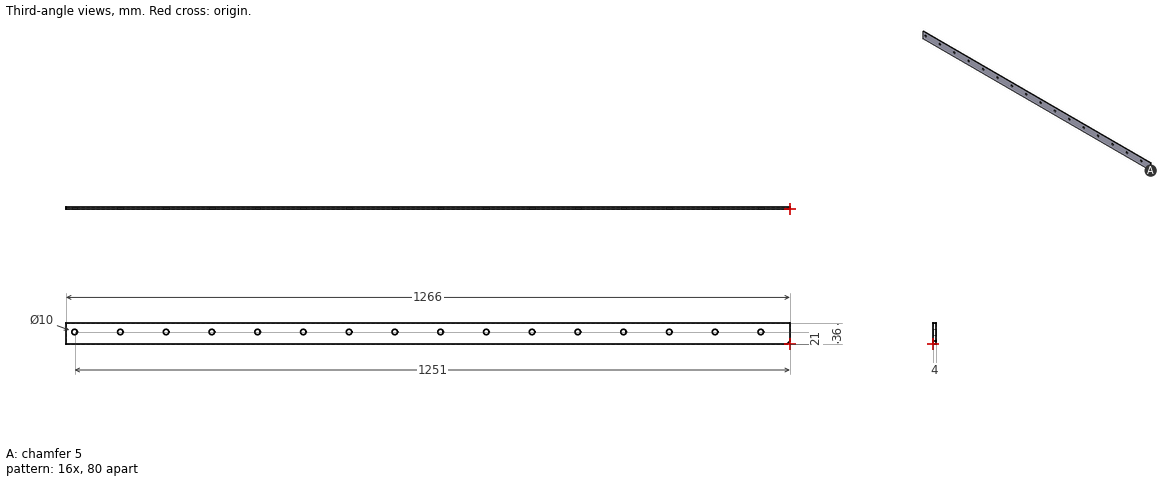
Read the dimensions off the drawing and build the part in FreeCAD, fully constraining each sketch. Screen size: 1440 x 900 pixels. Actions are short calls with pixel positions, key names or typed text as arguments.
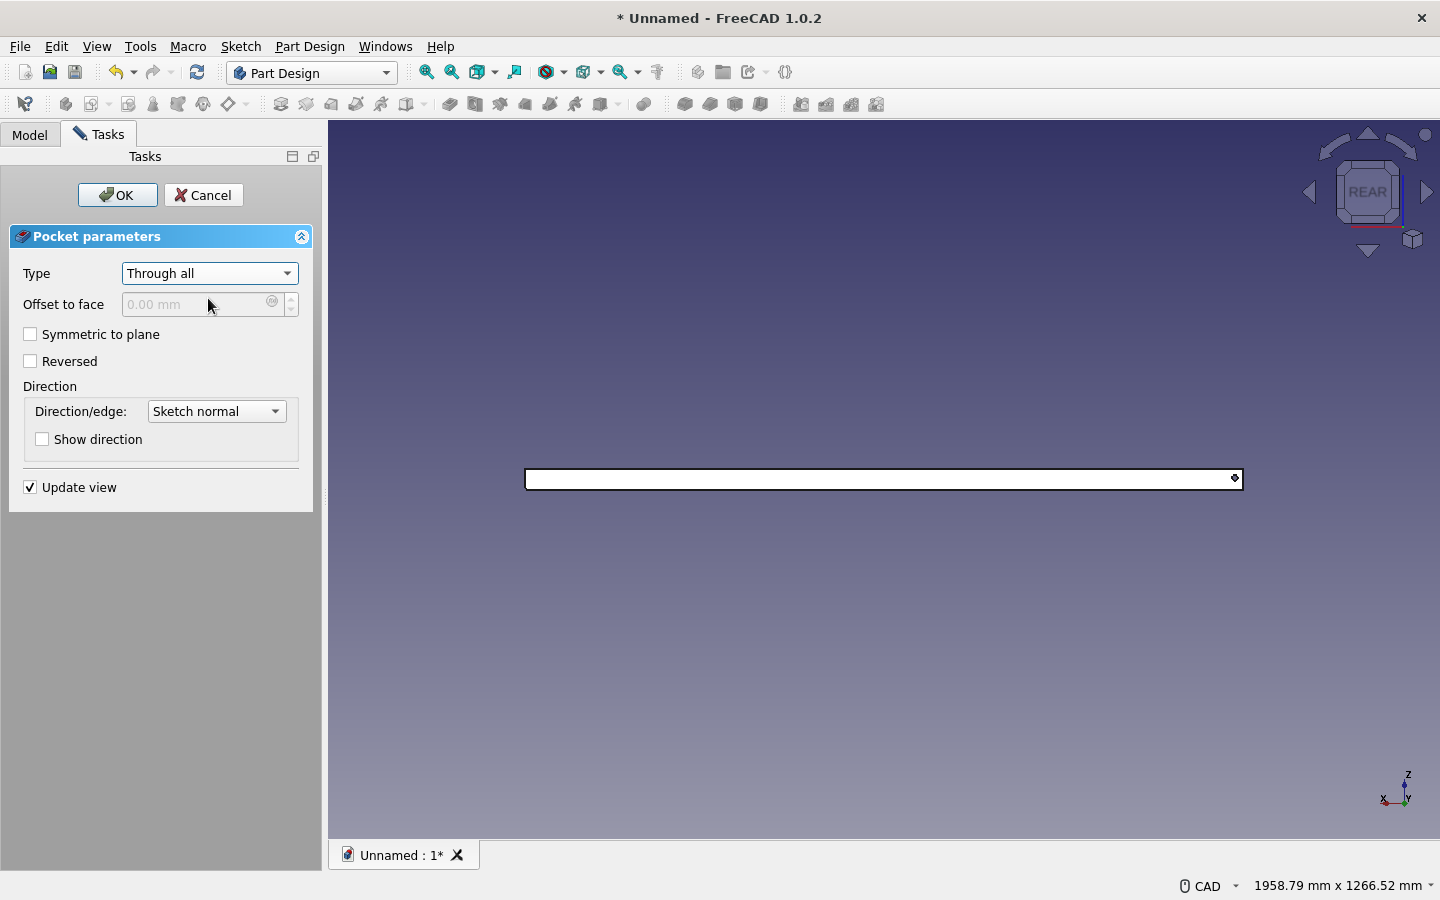
click(118, 195)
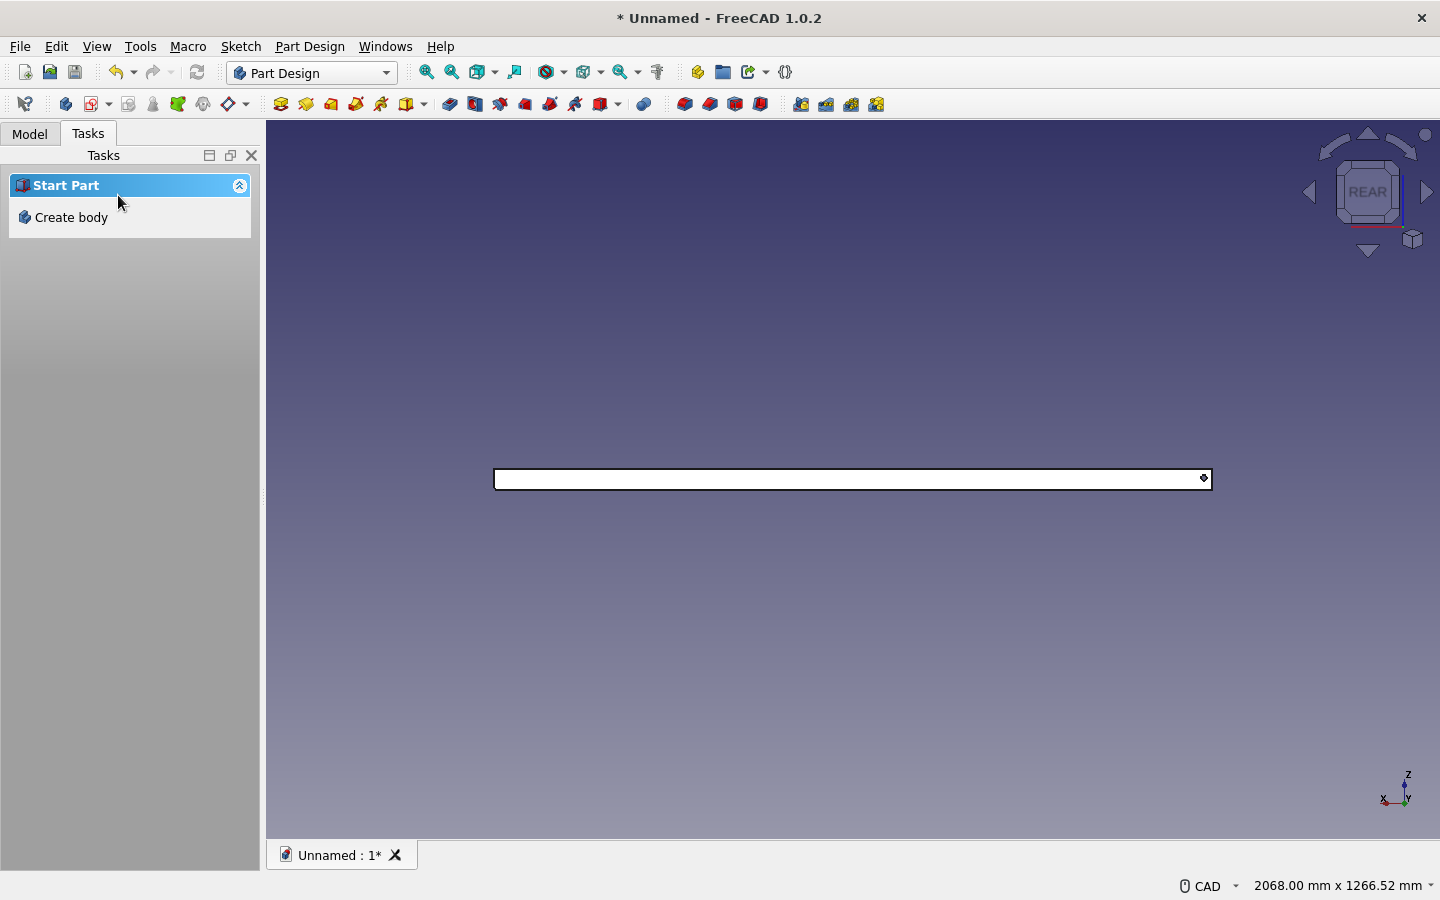
click(30, 134)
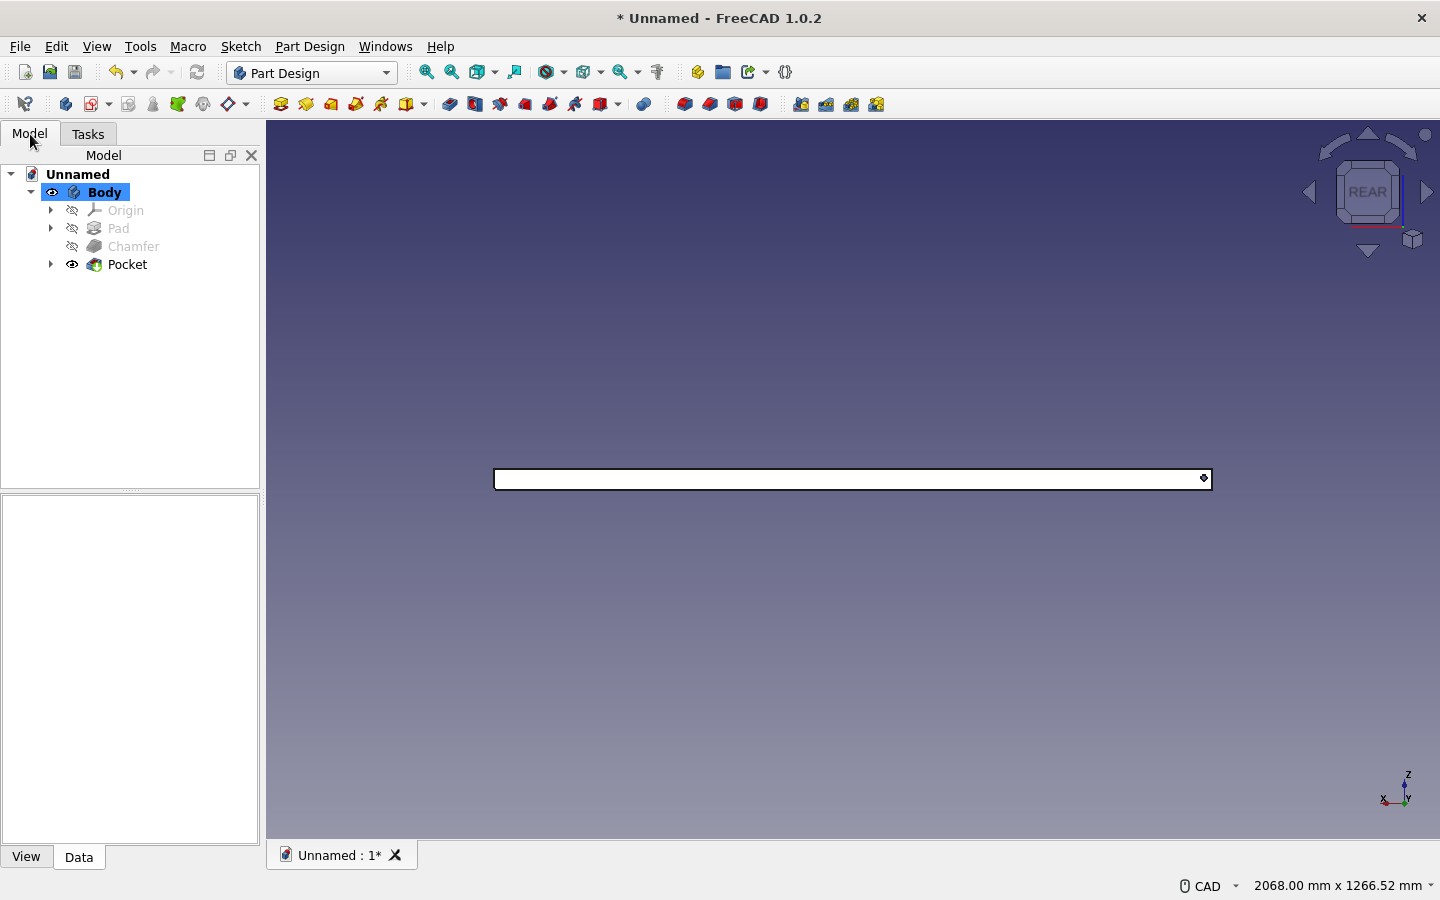
click(117, 264)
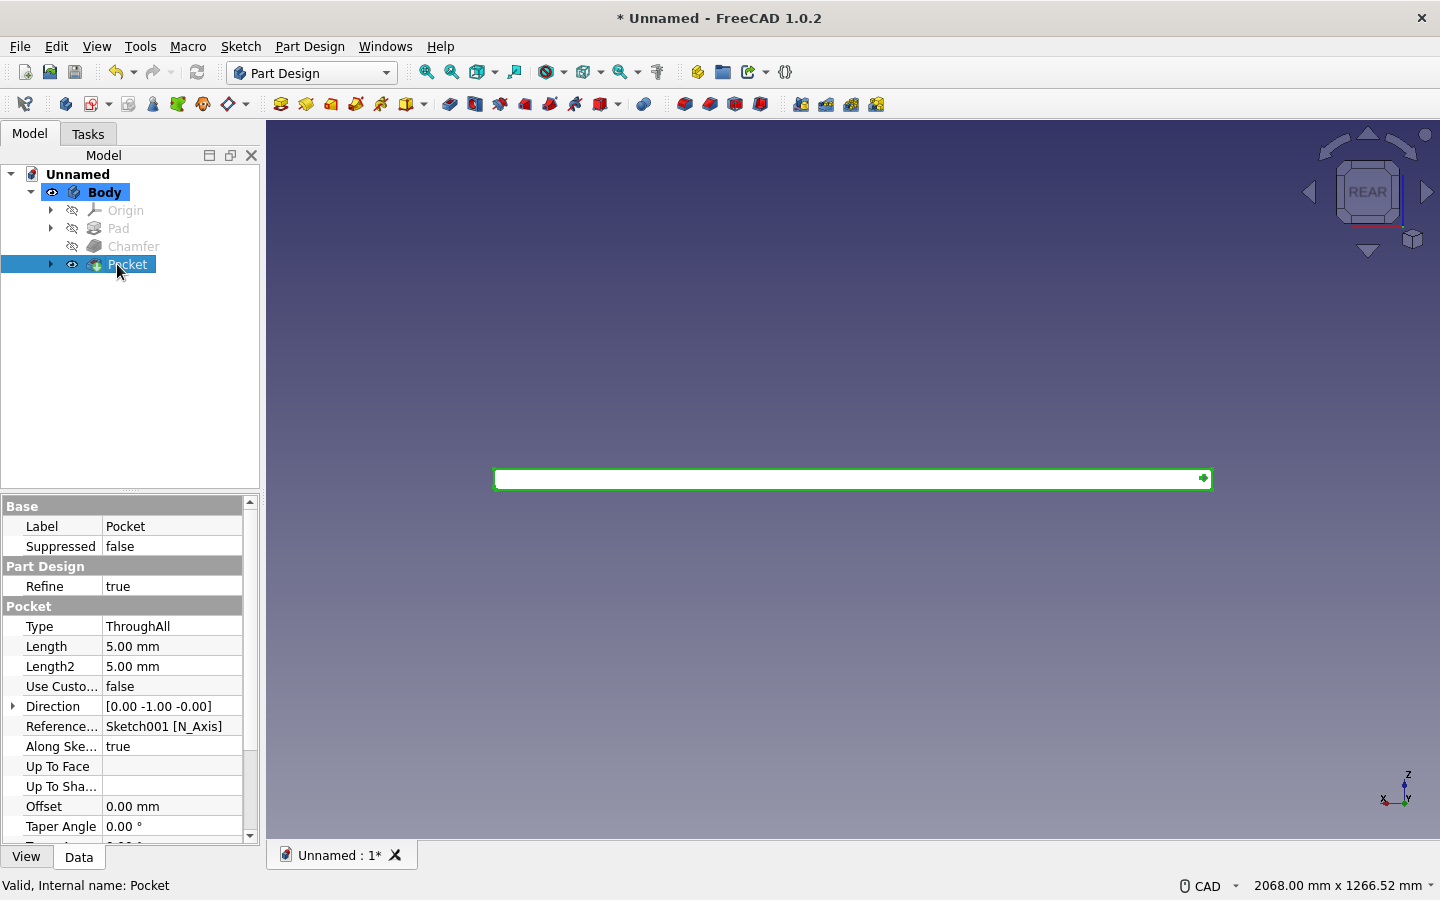
click(826, 104)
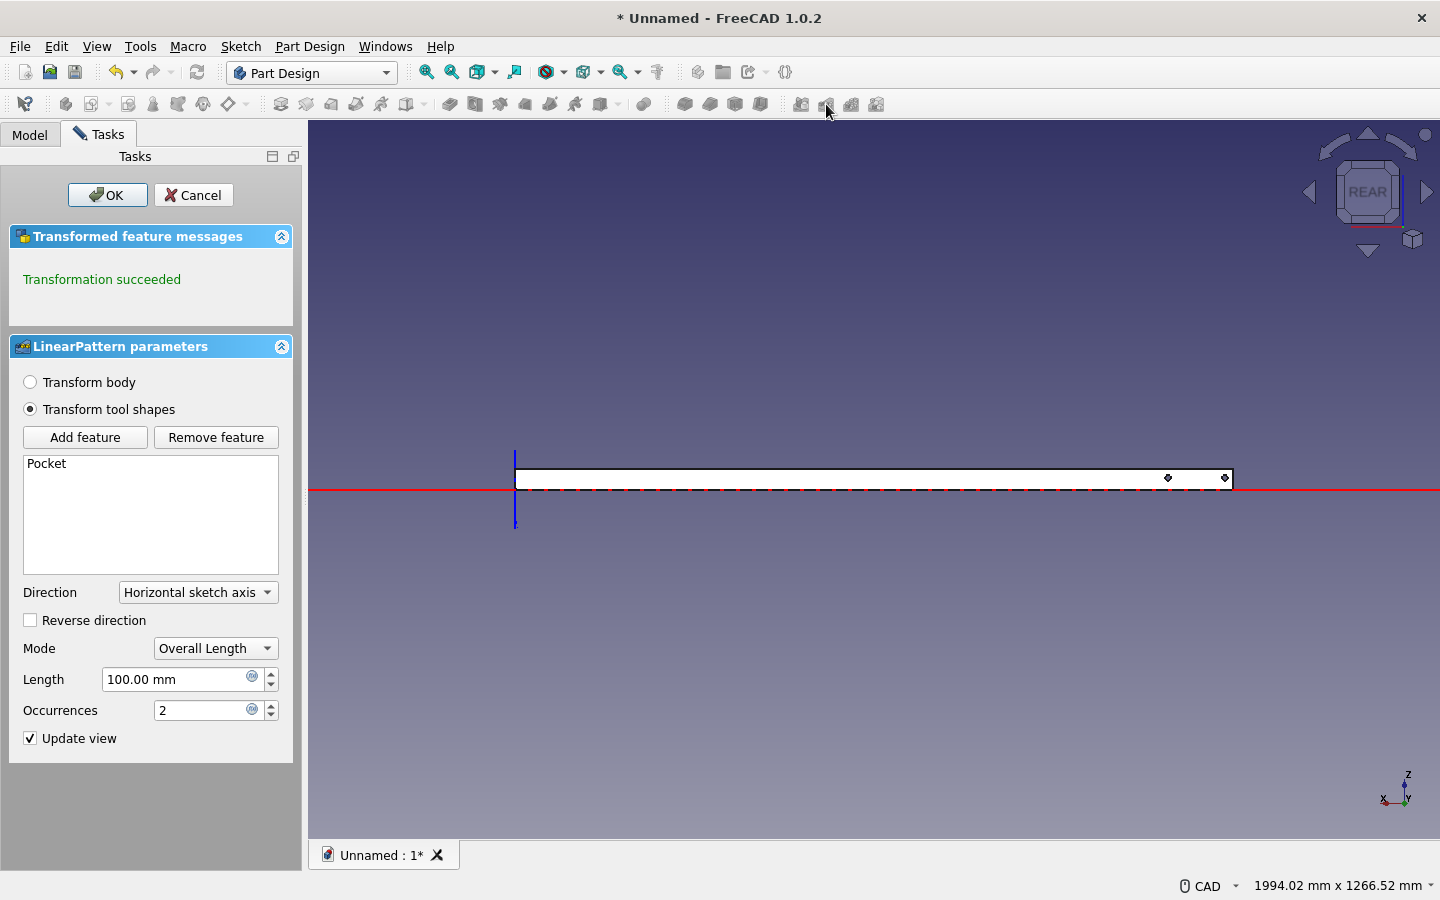
click(199, 592)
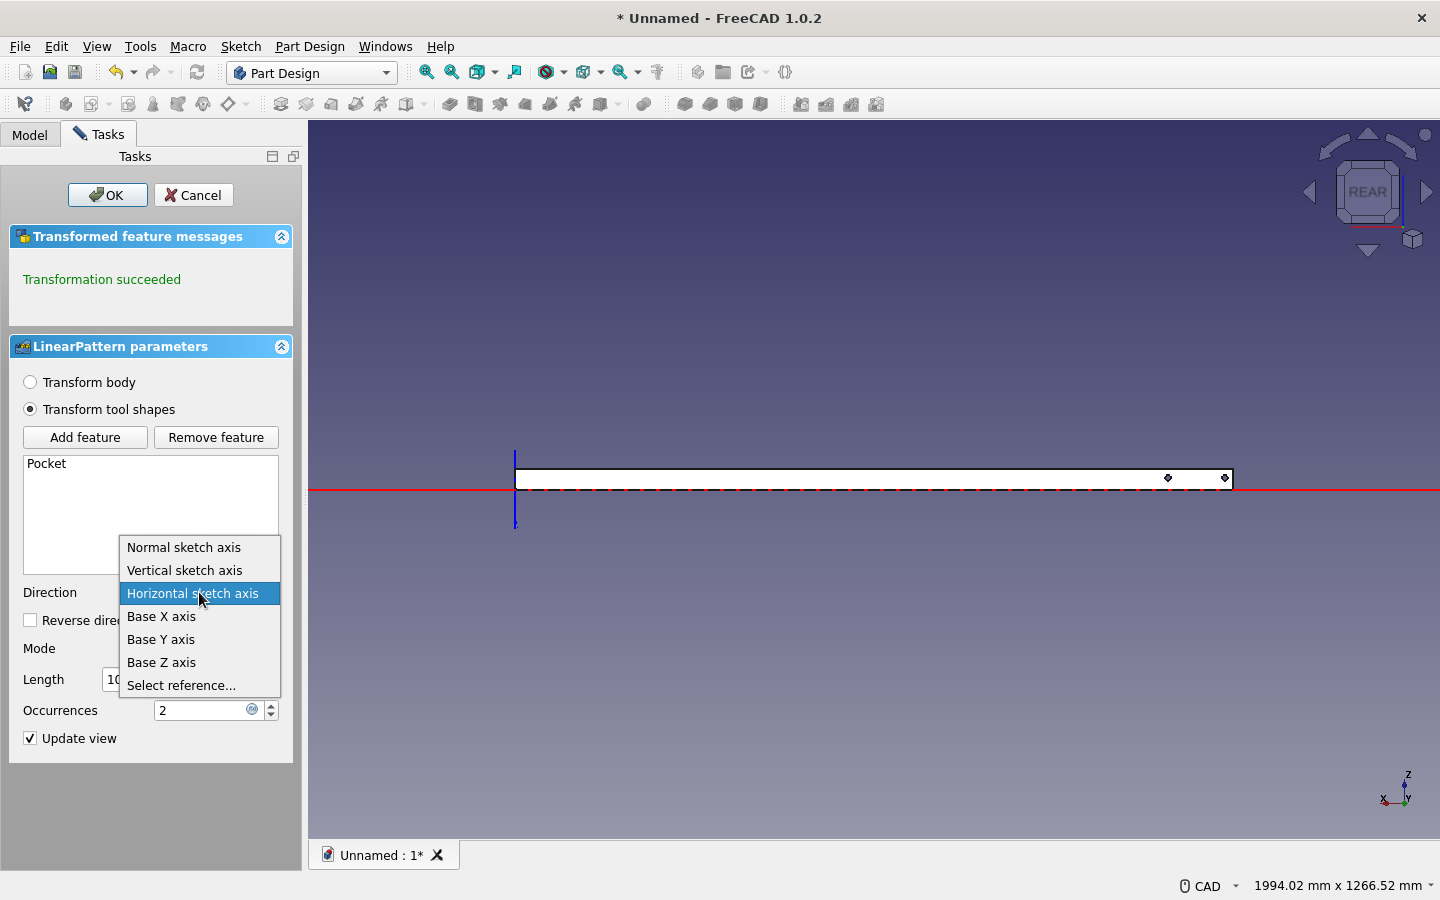
click(198, 616)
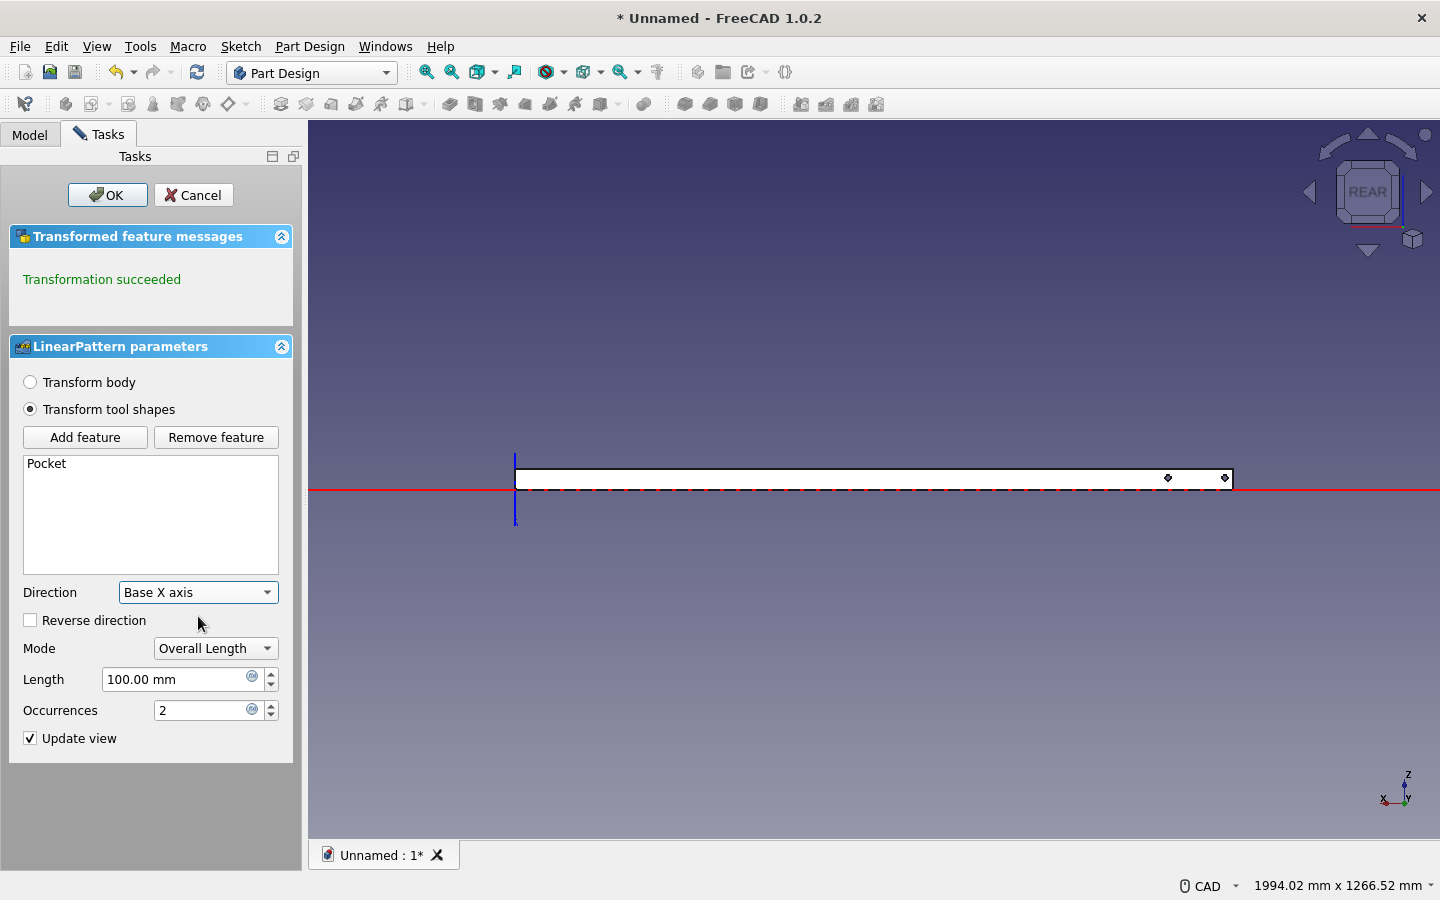
click(216, 648)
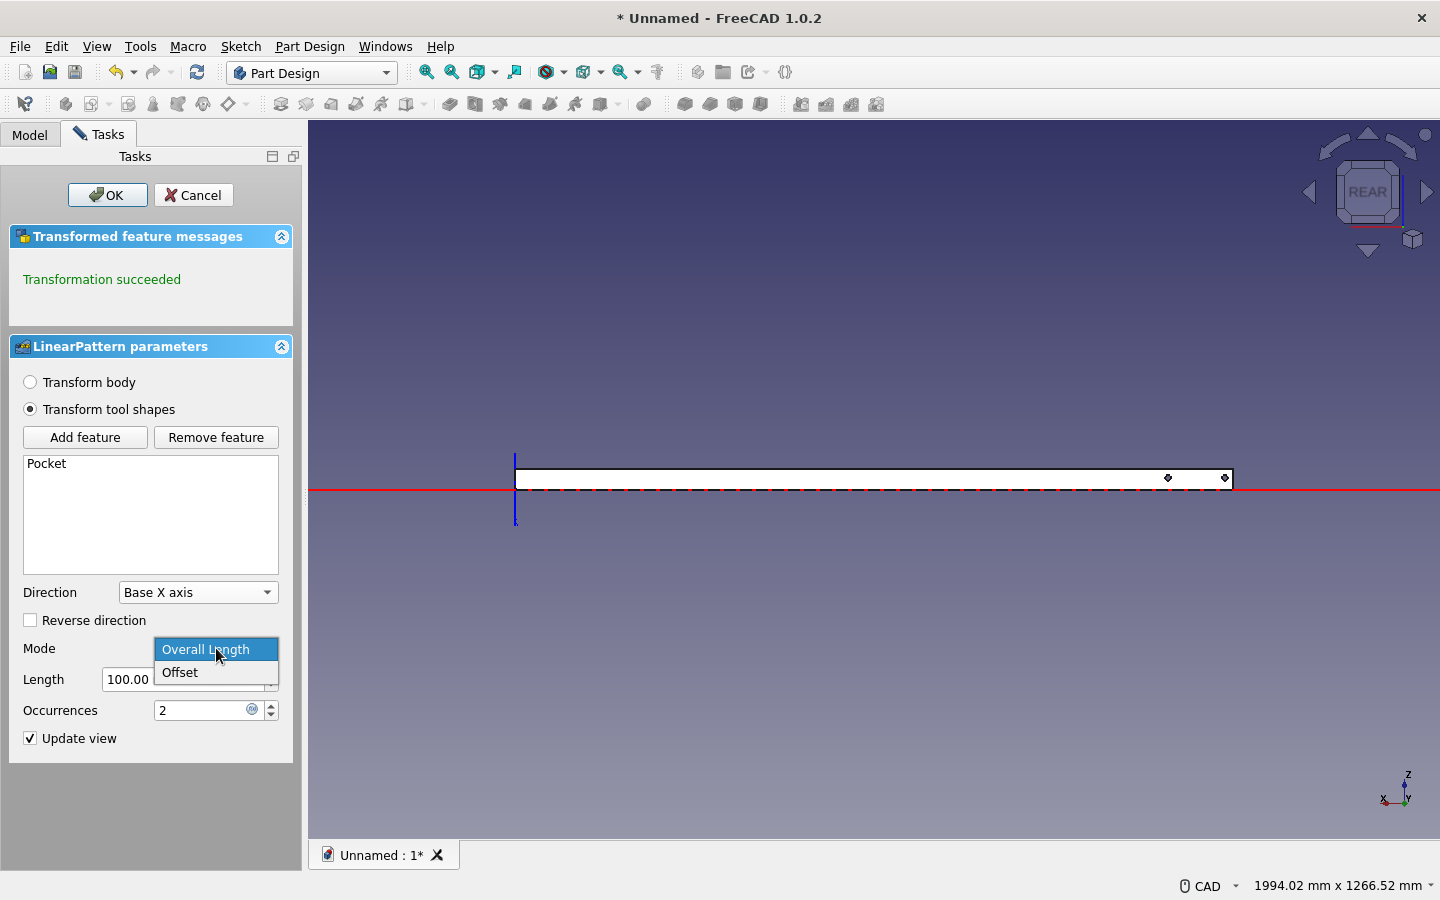
click(214, 672)